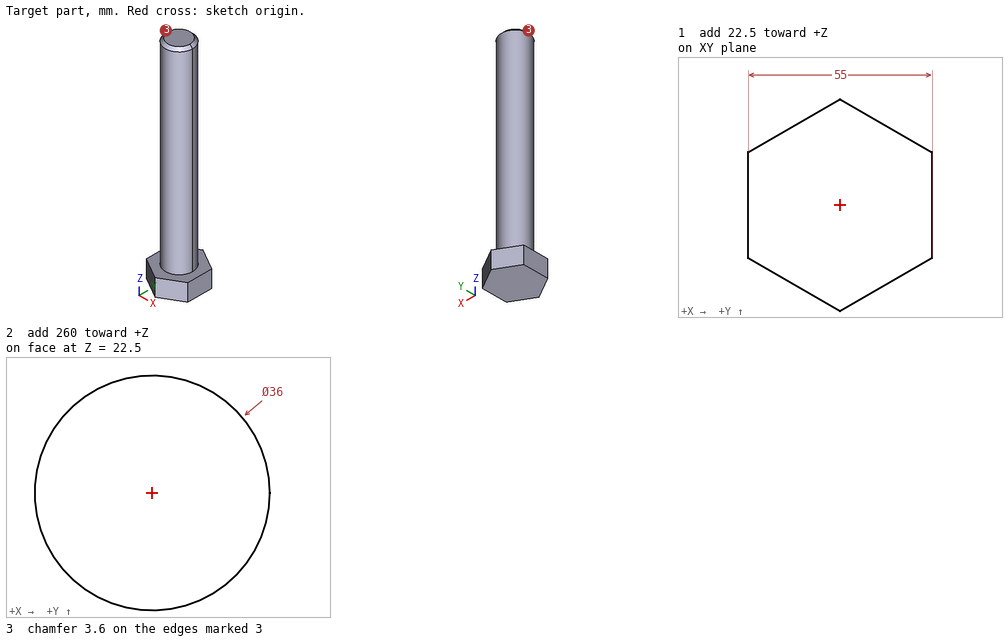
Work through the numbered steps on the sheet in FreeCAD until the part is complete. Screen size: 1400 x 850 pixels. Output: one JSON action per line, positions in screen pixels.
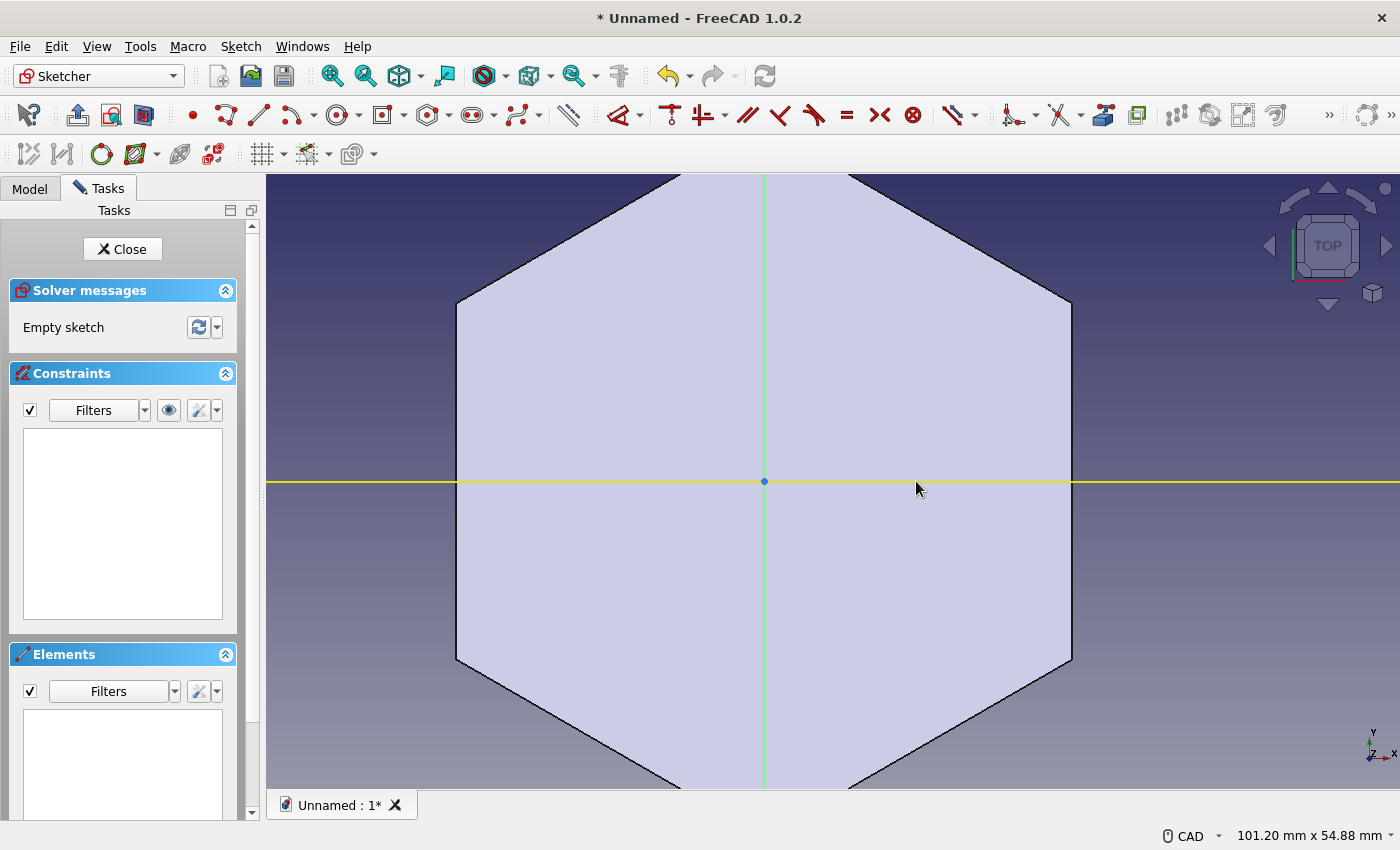
{"action": "left_click", "coordinate": [336, 116]}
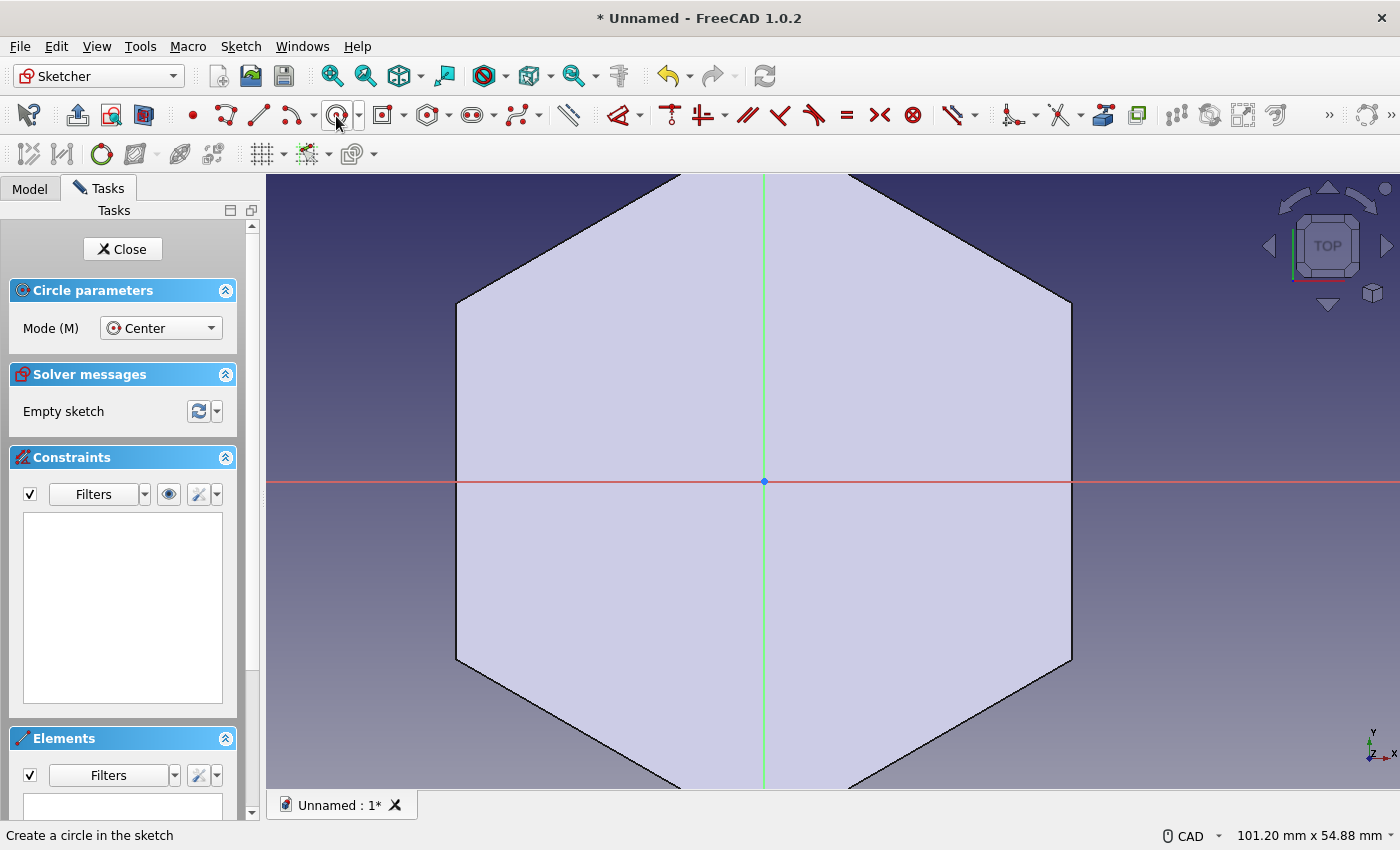
{"action": "left_click", "coordinate": [764, 482]}
{"action": "mouse_move", "coordinate": [907, 339]}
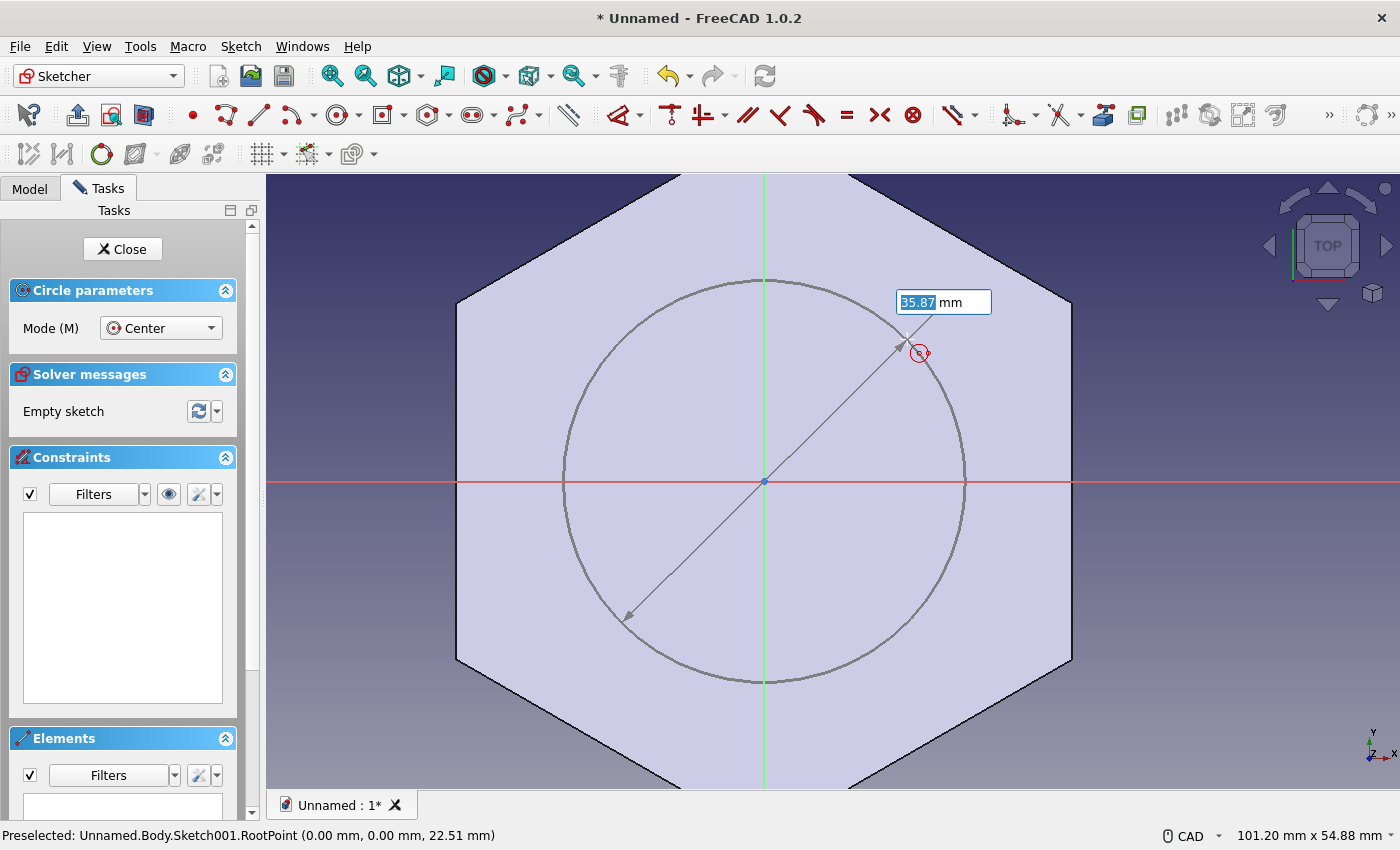
{"action": "type", "text": "36"}
{"action": "key", "text": "Return"}
{"action": "key", "text": "Escape"}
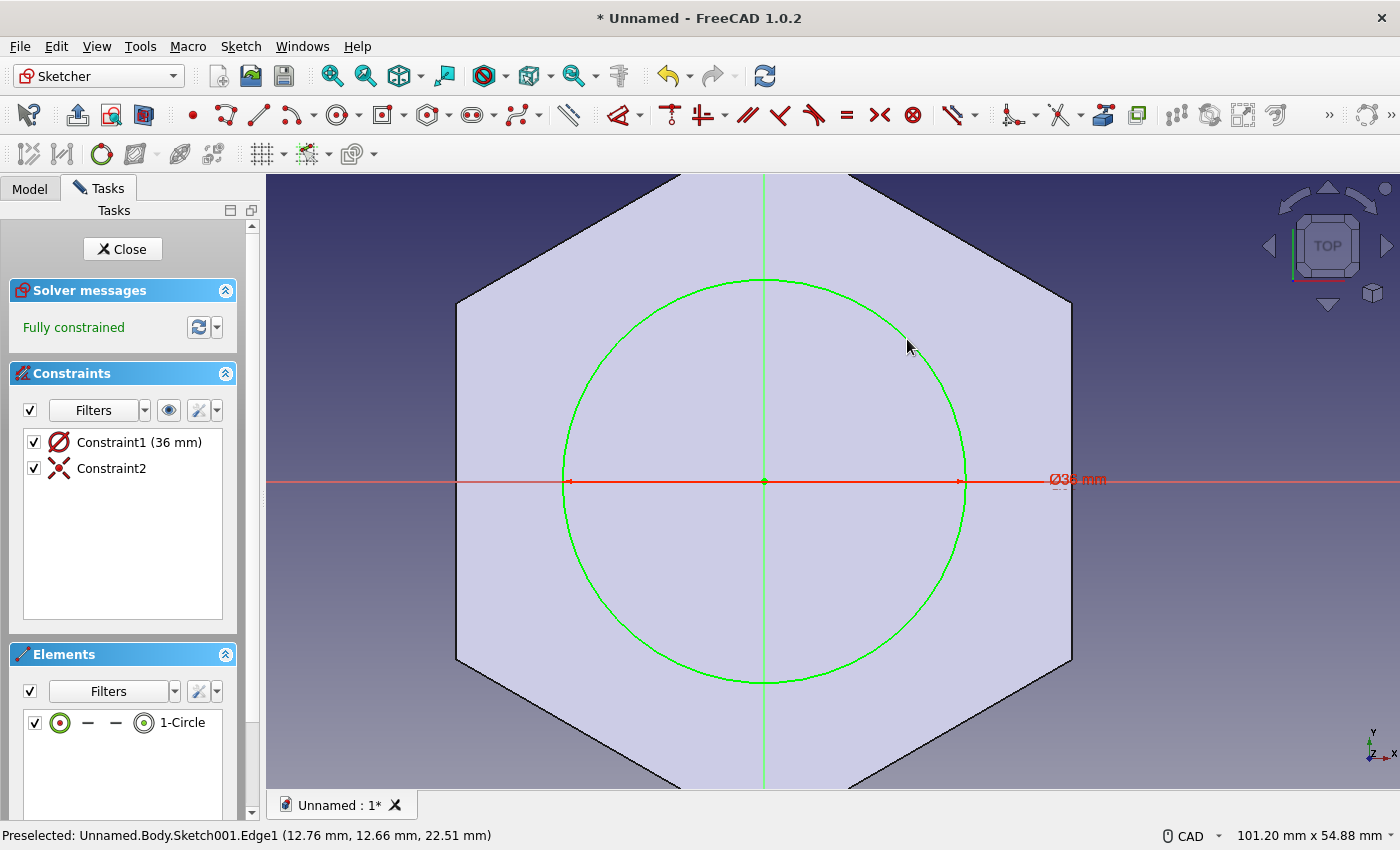
{"action": "left_click", "coordinate": [123, 249]}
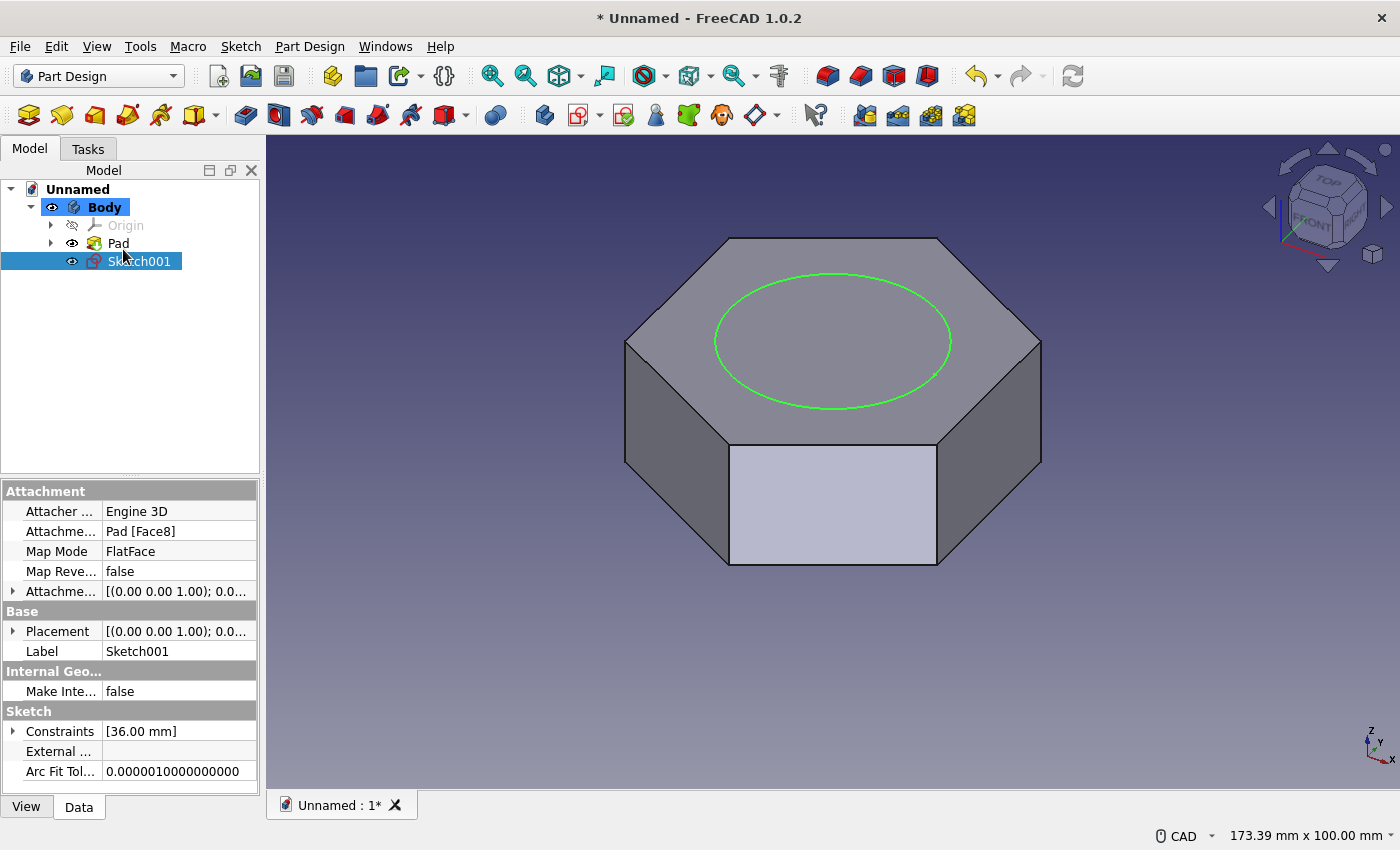
{"action": "left_click", "coordinate": [29, 116]}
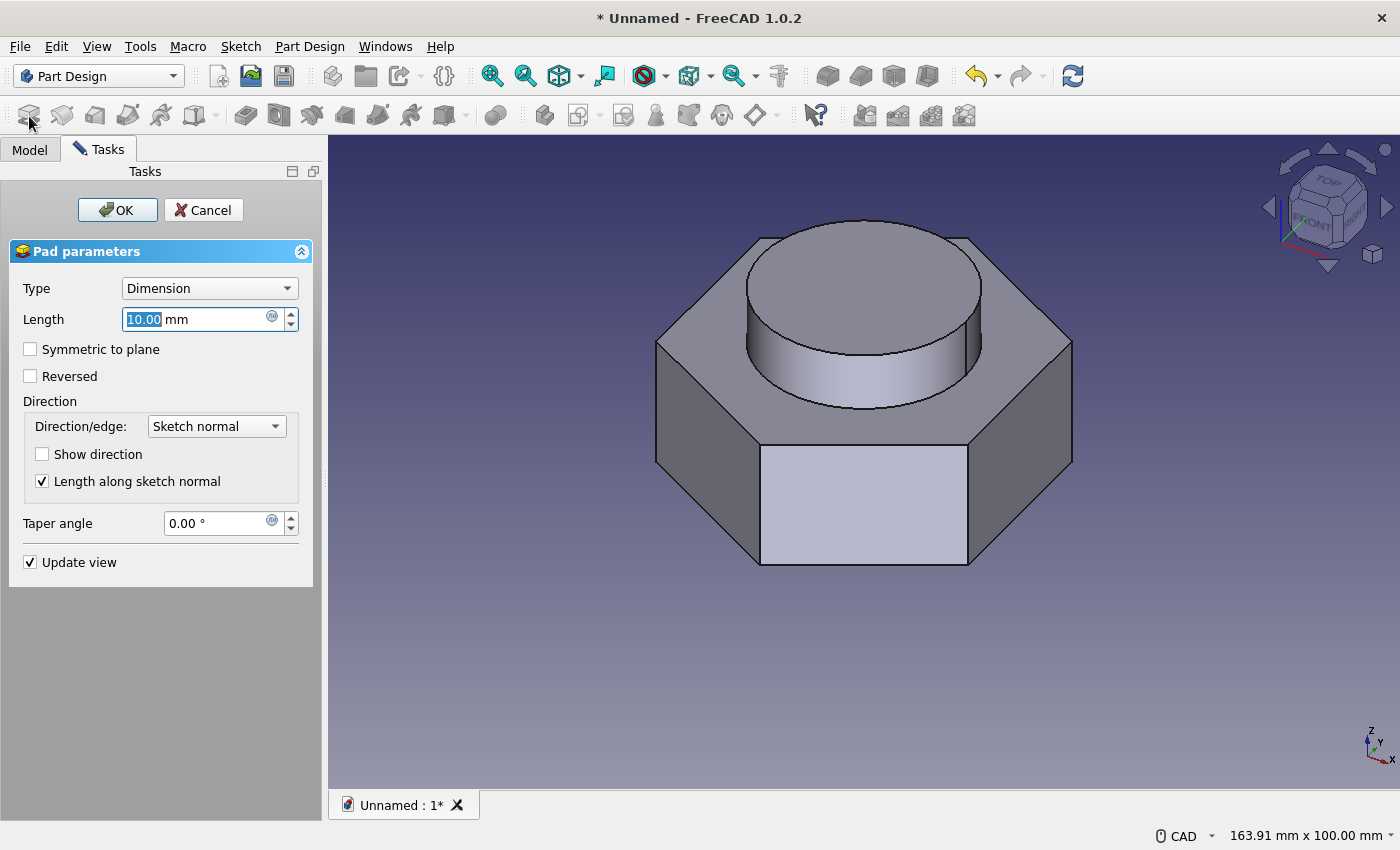
{"action": "type", "text": "260"}
{"action": "key", "text": "Tab"}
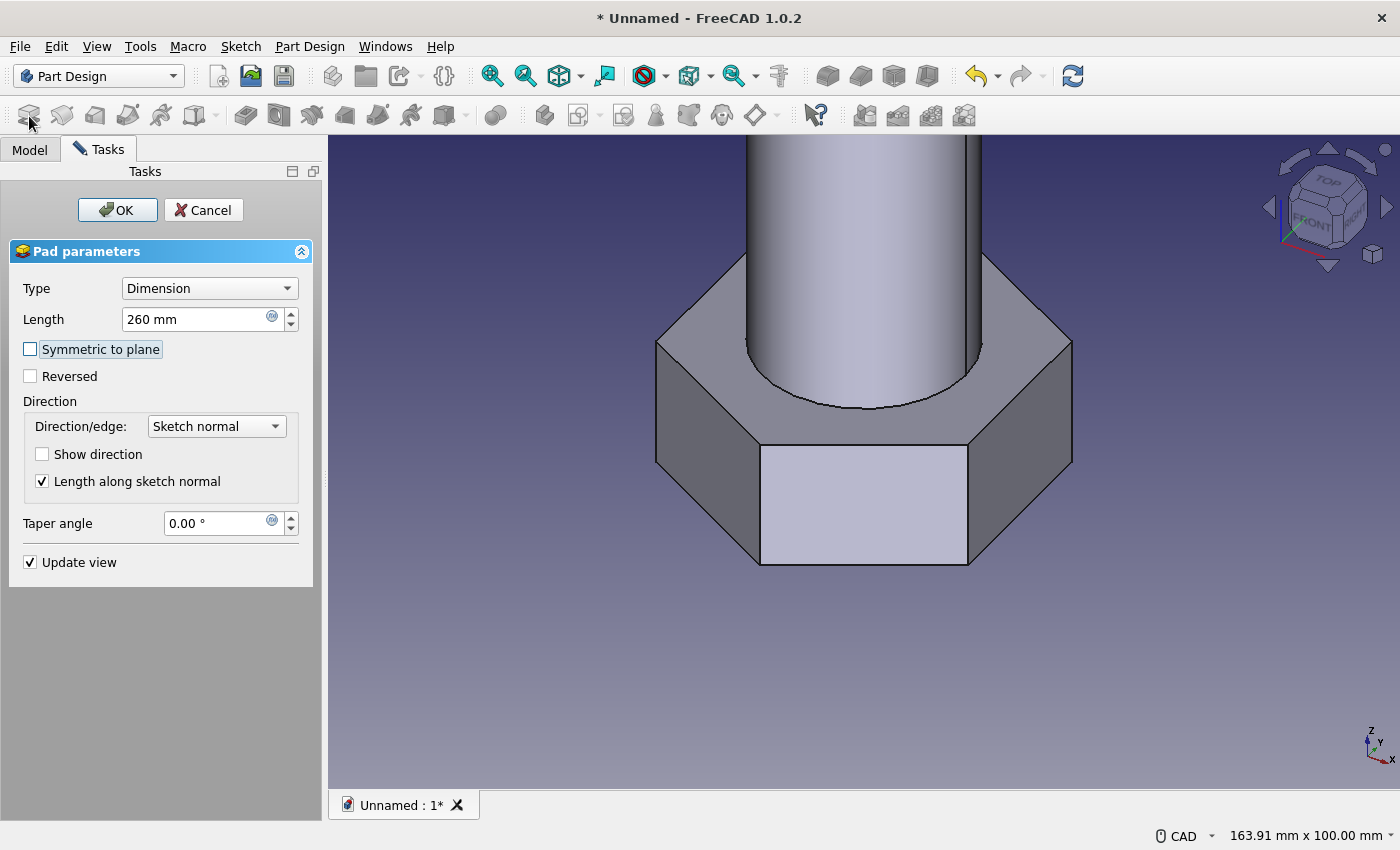
{"action": "left_click", "coordinate": [118, 210]}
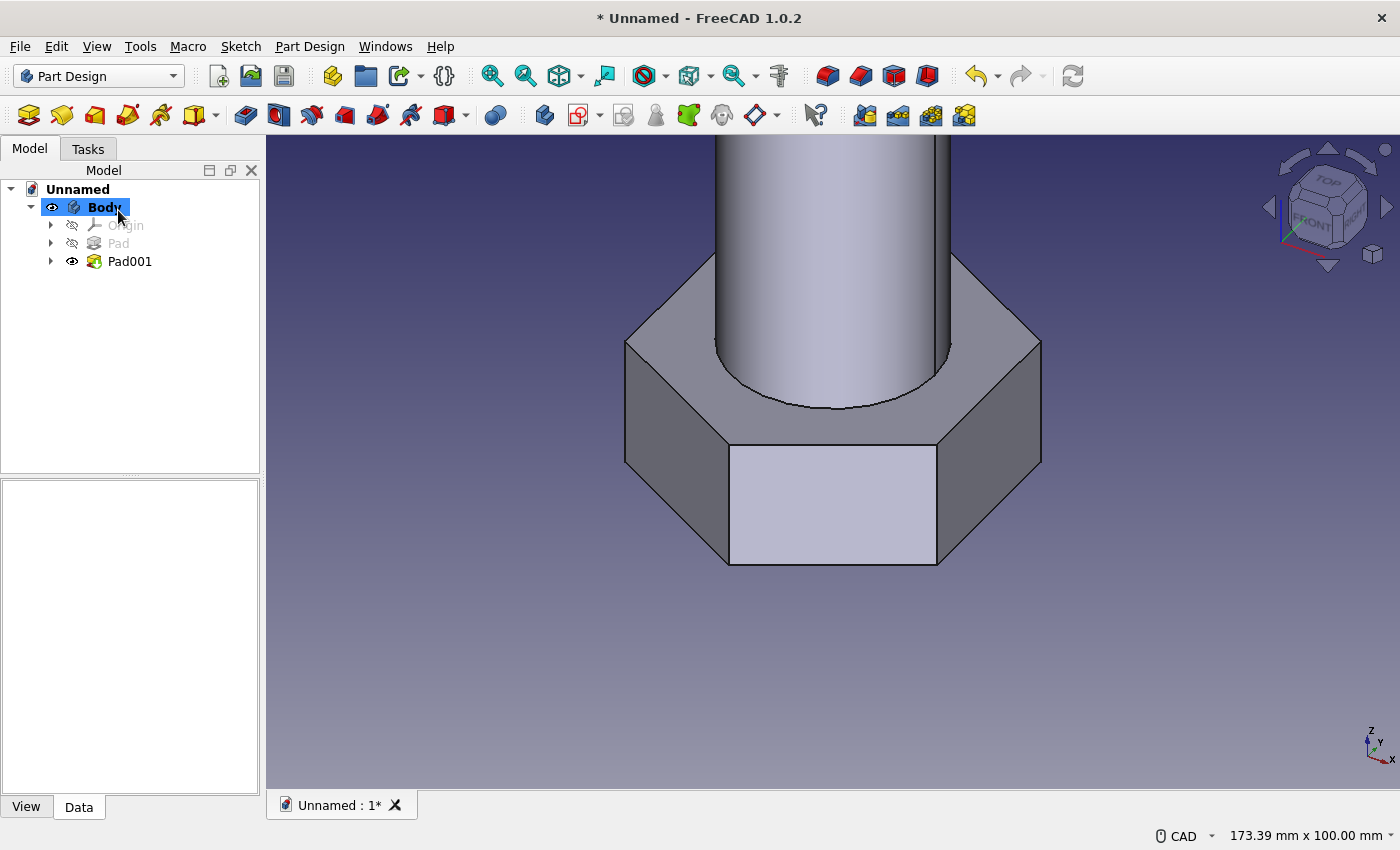
{"action": "left_click", "coordinate": [493, 76]}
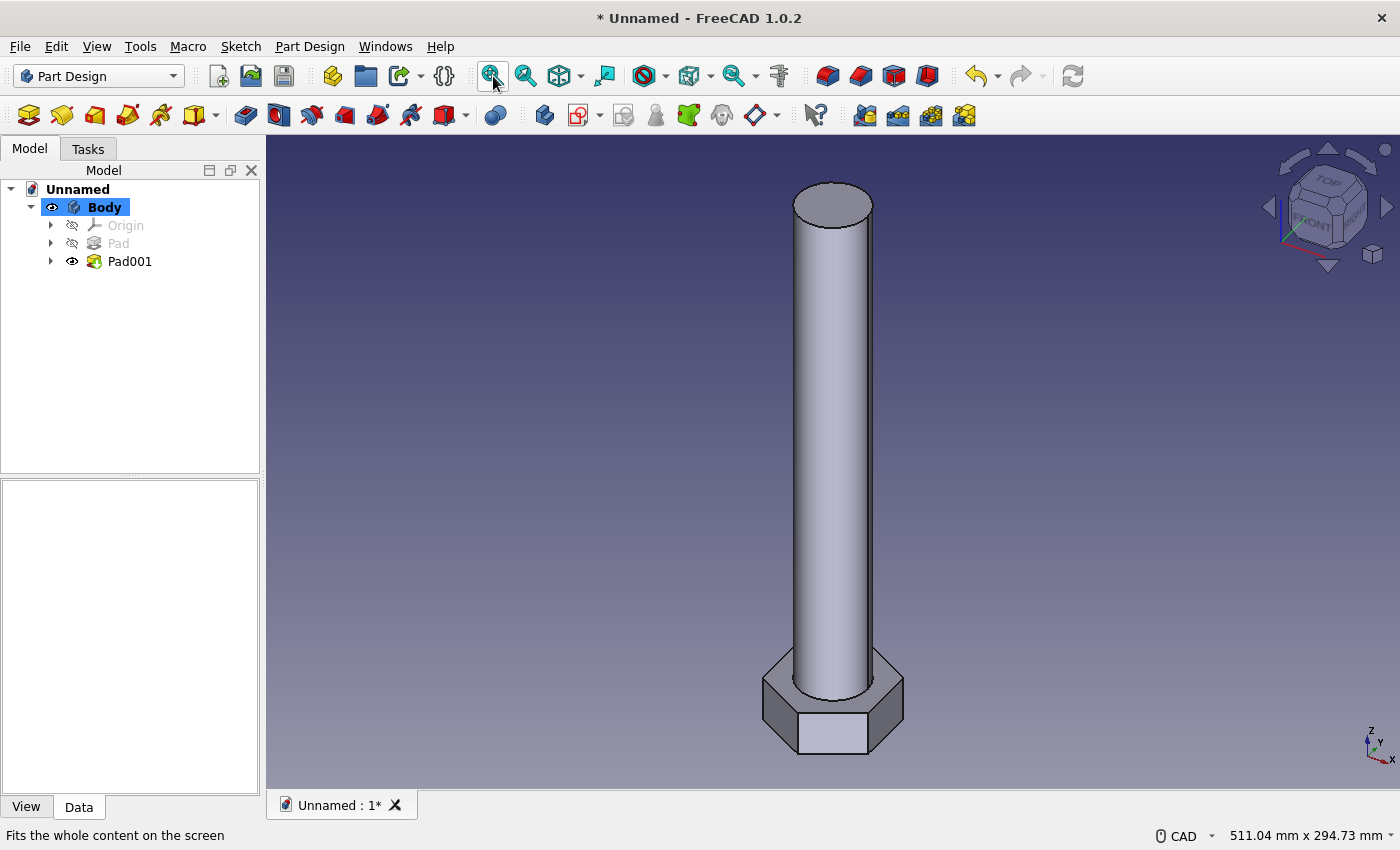
{"action": "left_click", "coordinate": [793, 207]}